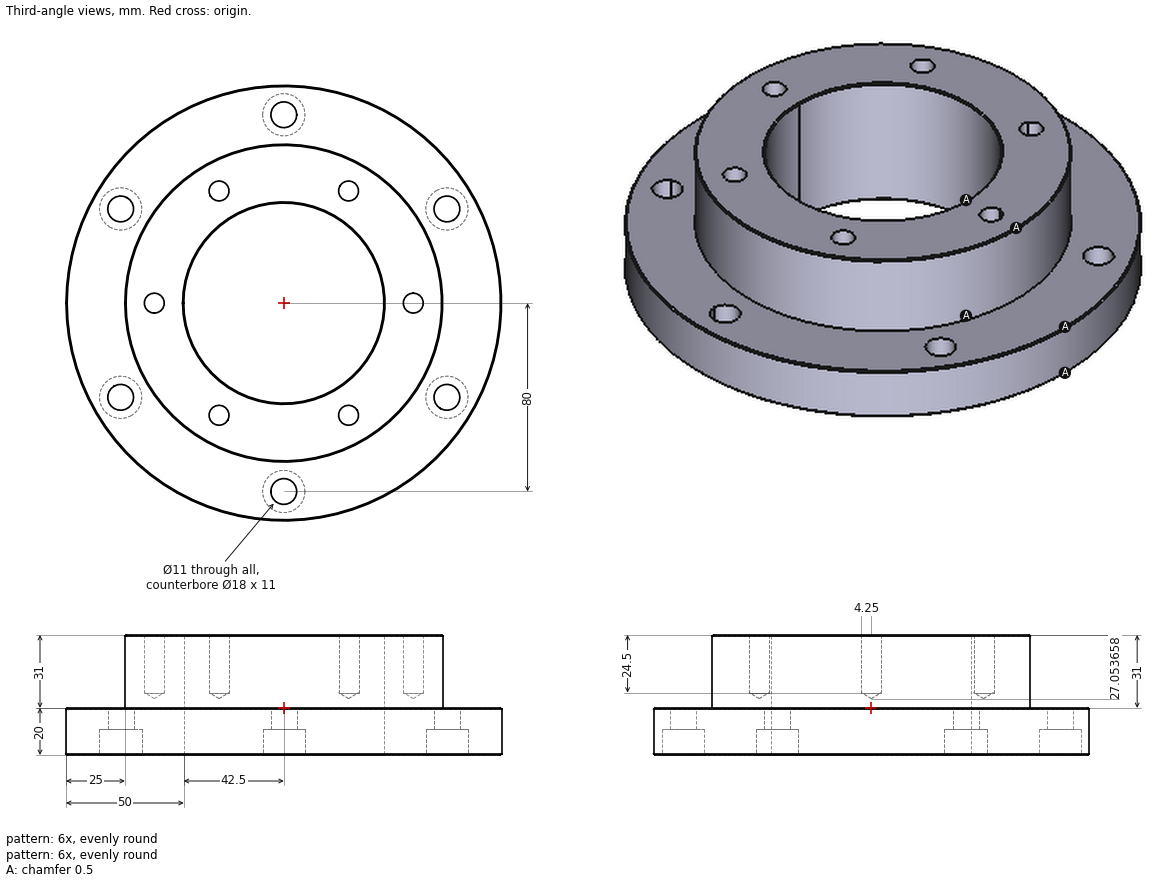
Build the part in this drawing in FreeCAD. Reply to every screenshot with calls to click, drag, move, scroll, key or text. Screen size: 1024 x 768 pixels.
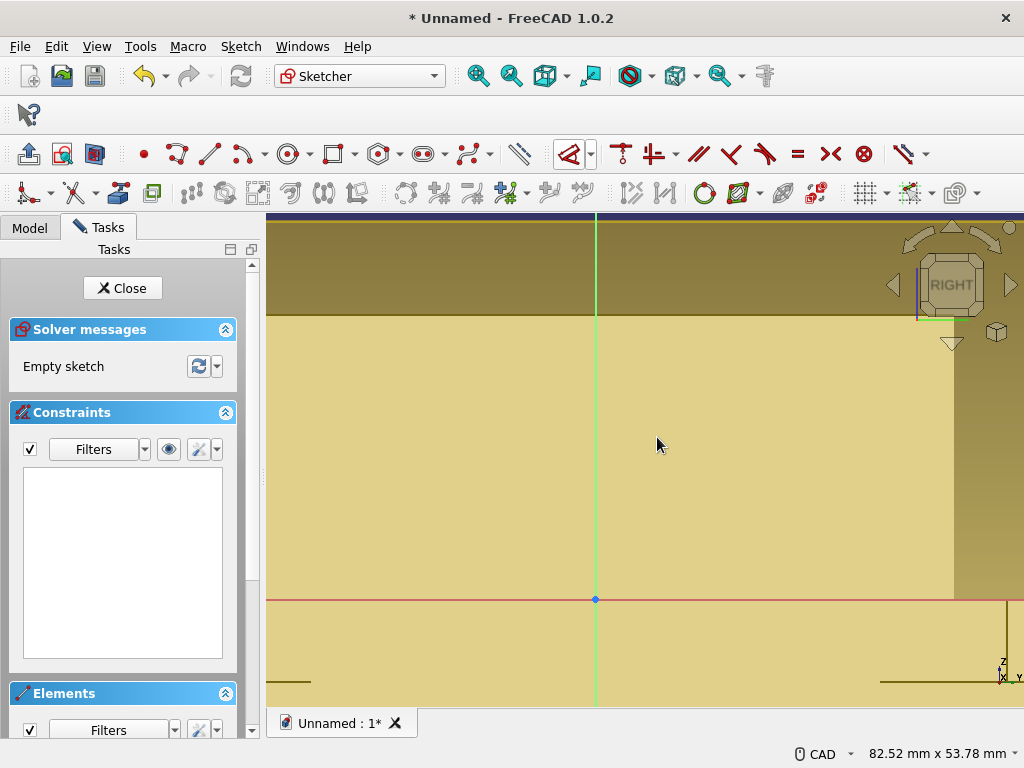
click(177, 154)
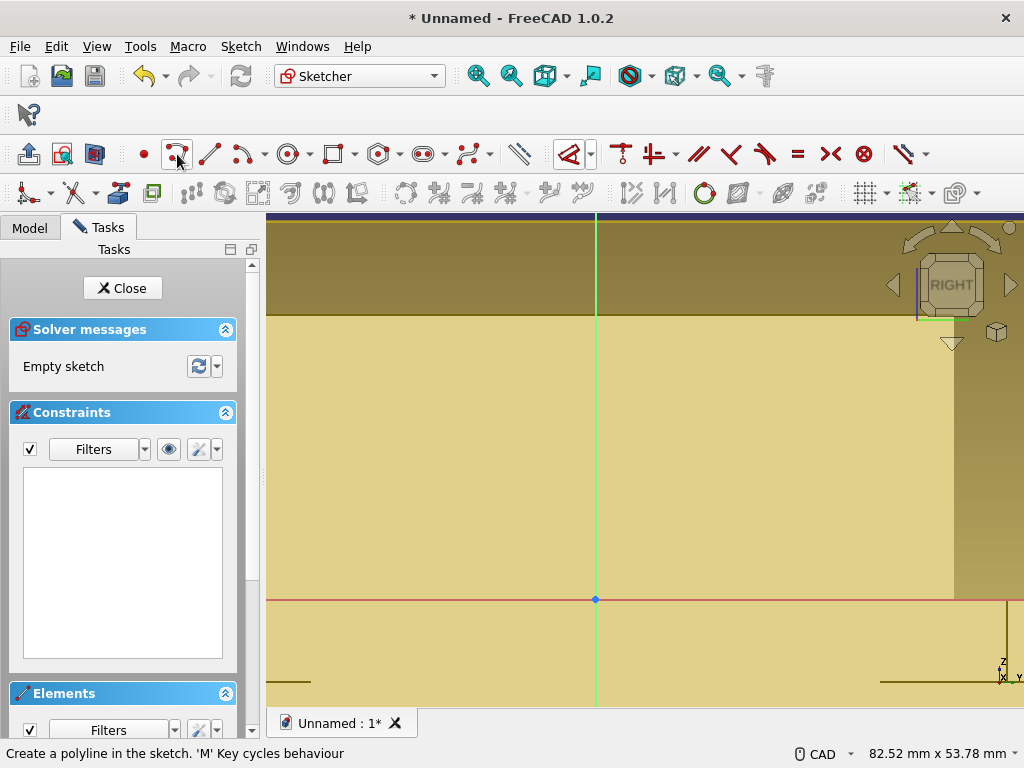
click(596, 563)
click(587, 315)
click(556, 315)
click(556, 540)
click(596, 564)
key(Escape)
key(Escape)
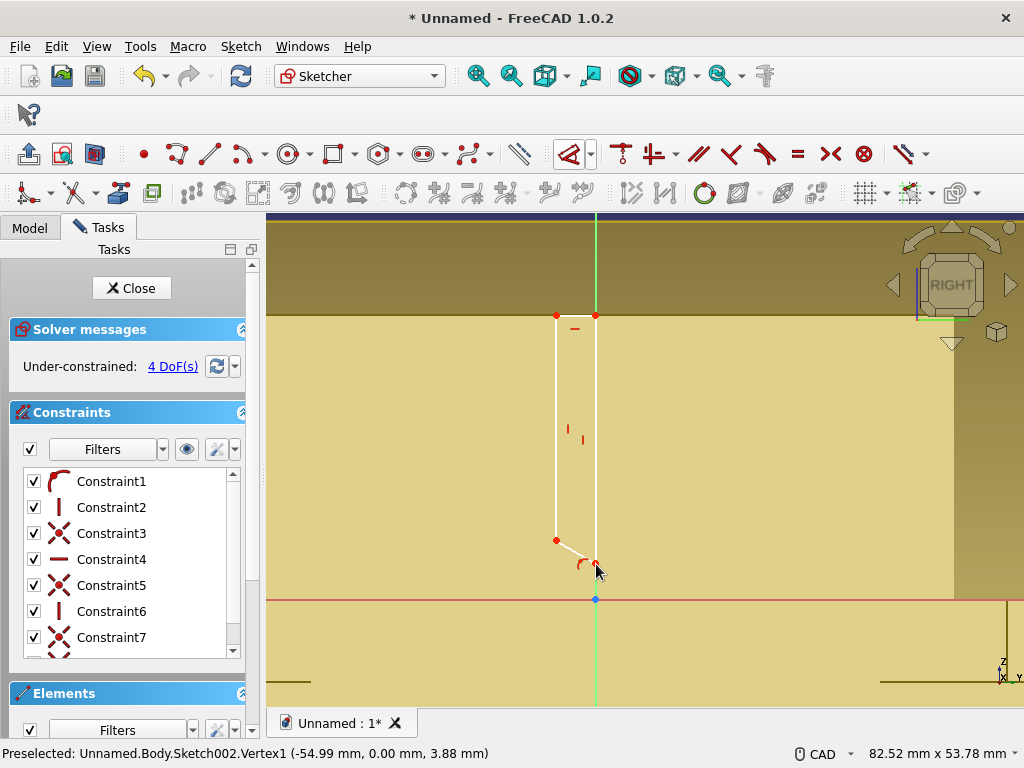
click(596, 316)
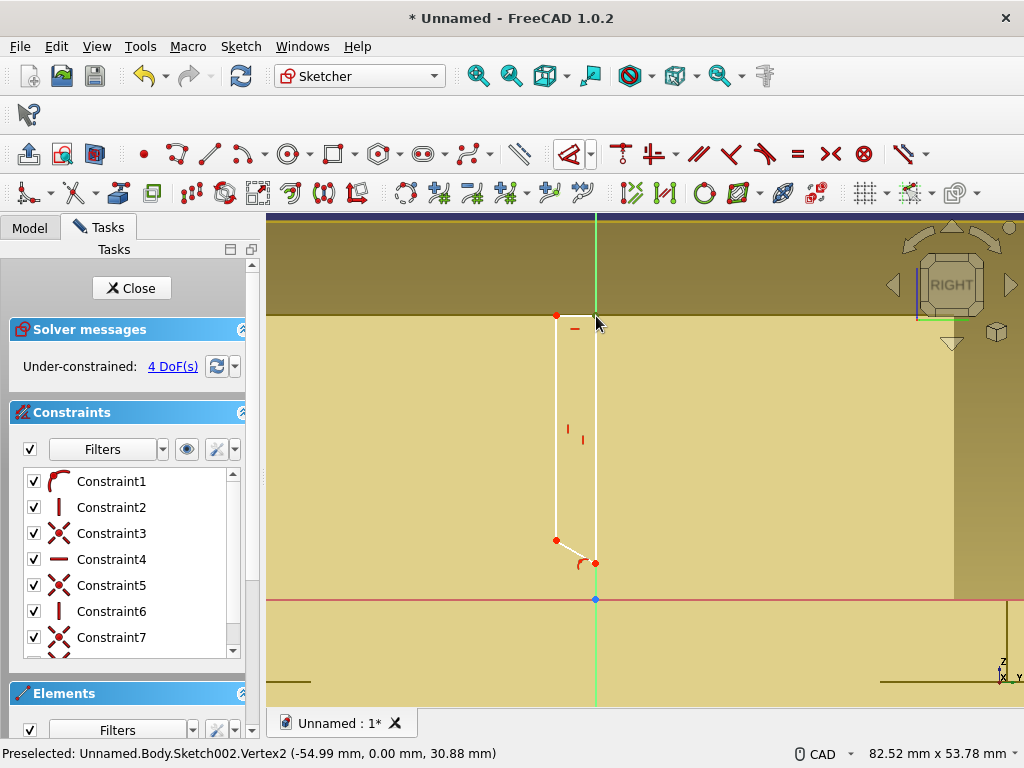
click(590, 154)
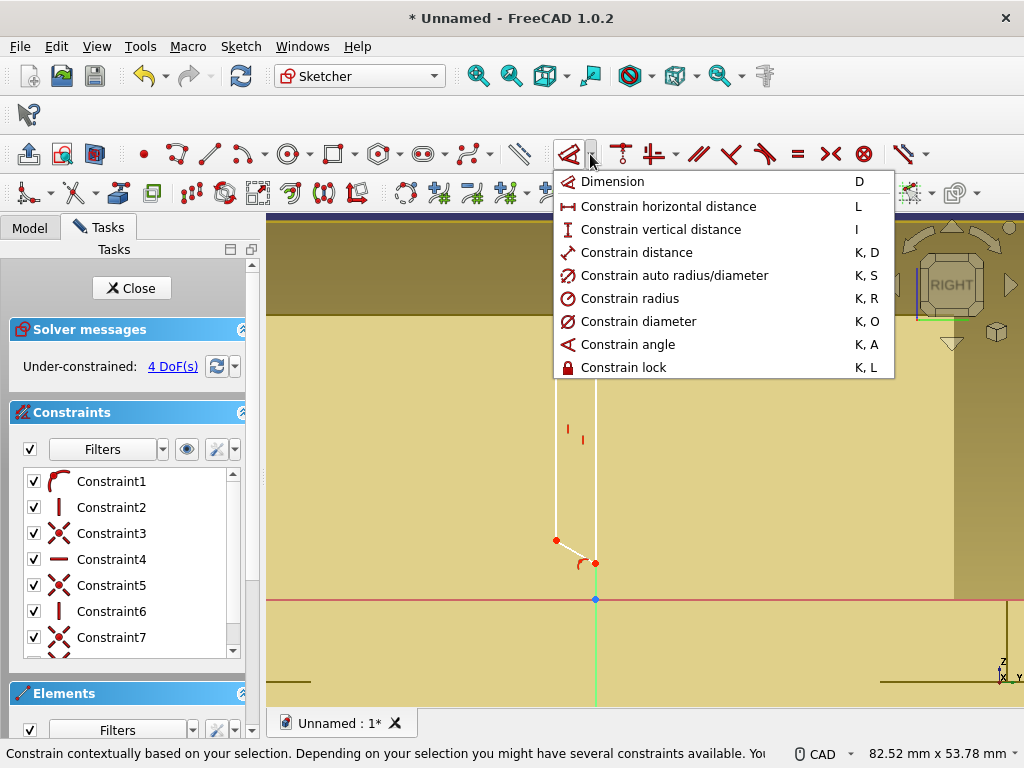
click(724, 230)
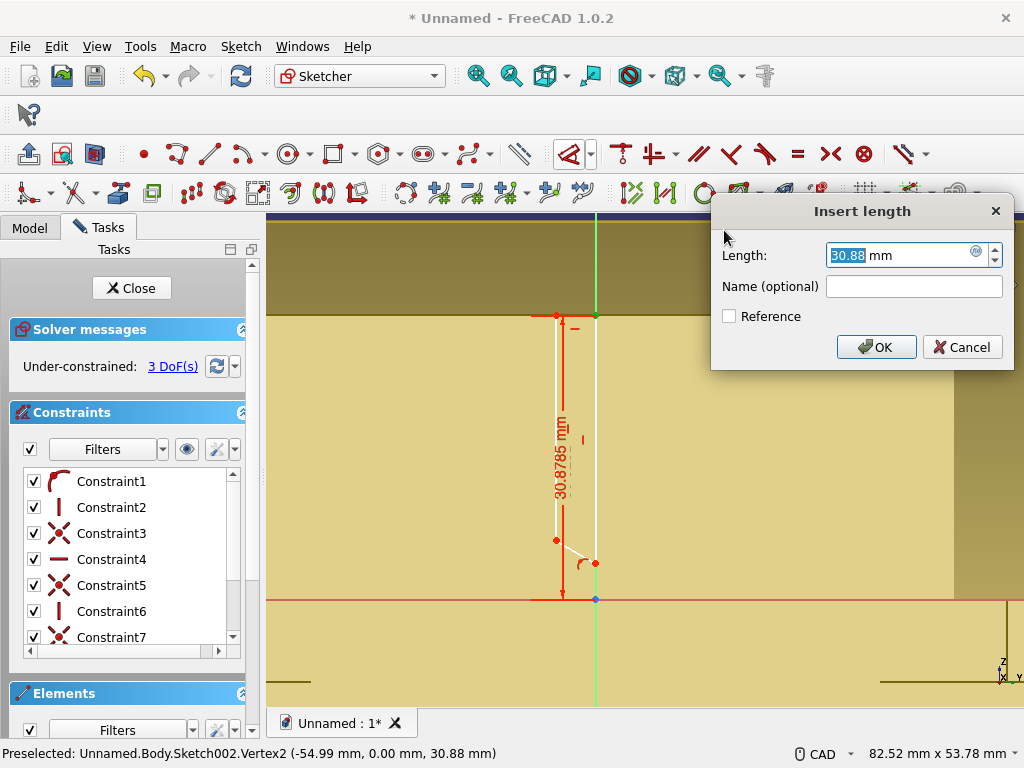
text(31)
key(Return)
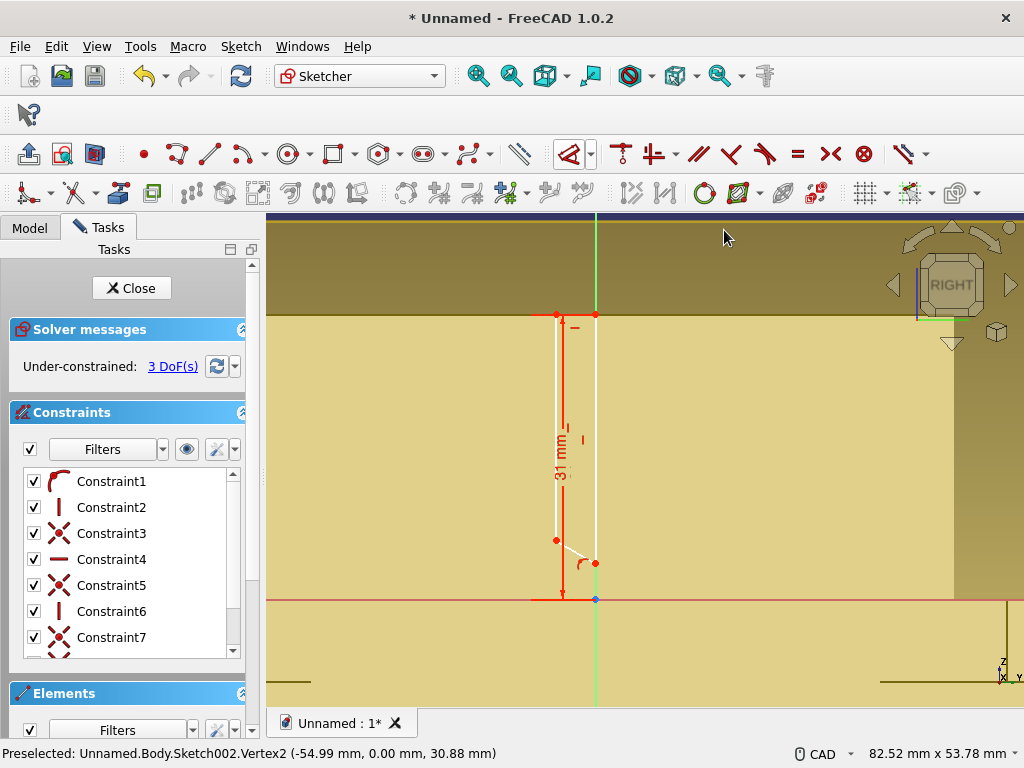
click(584, 315)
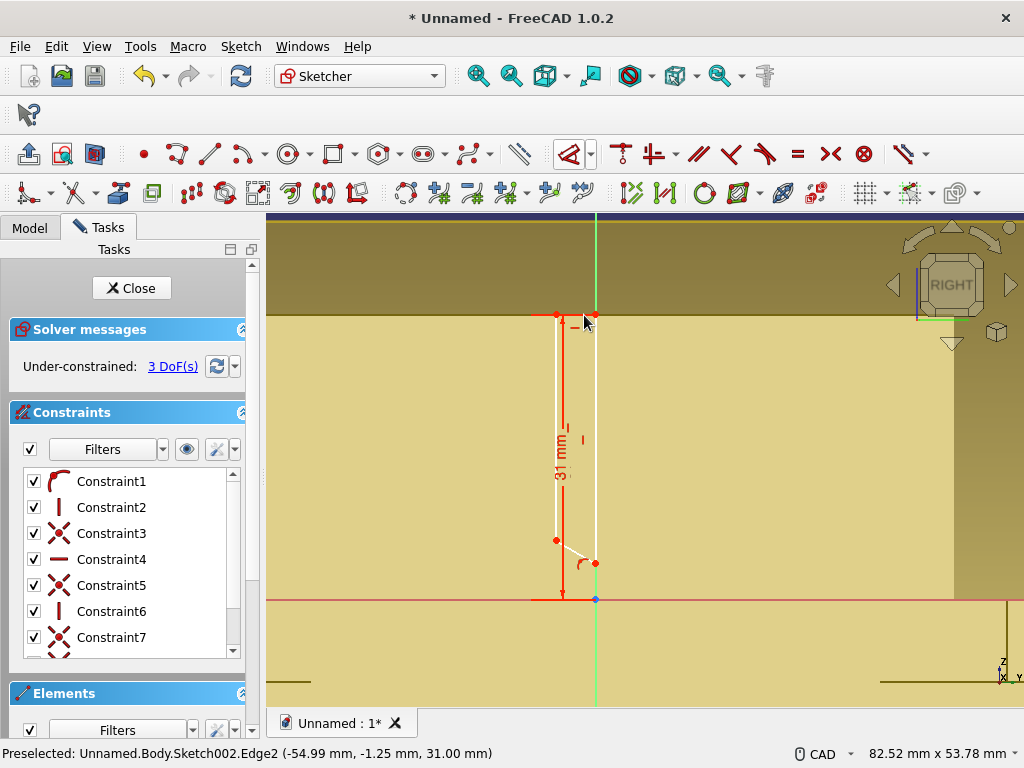
click(590, 154)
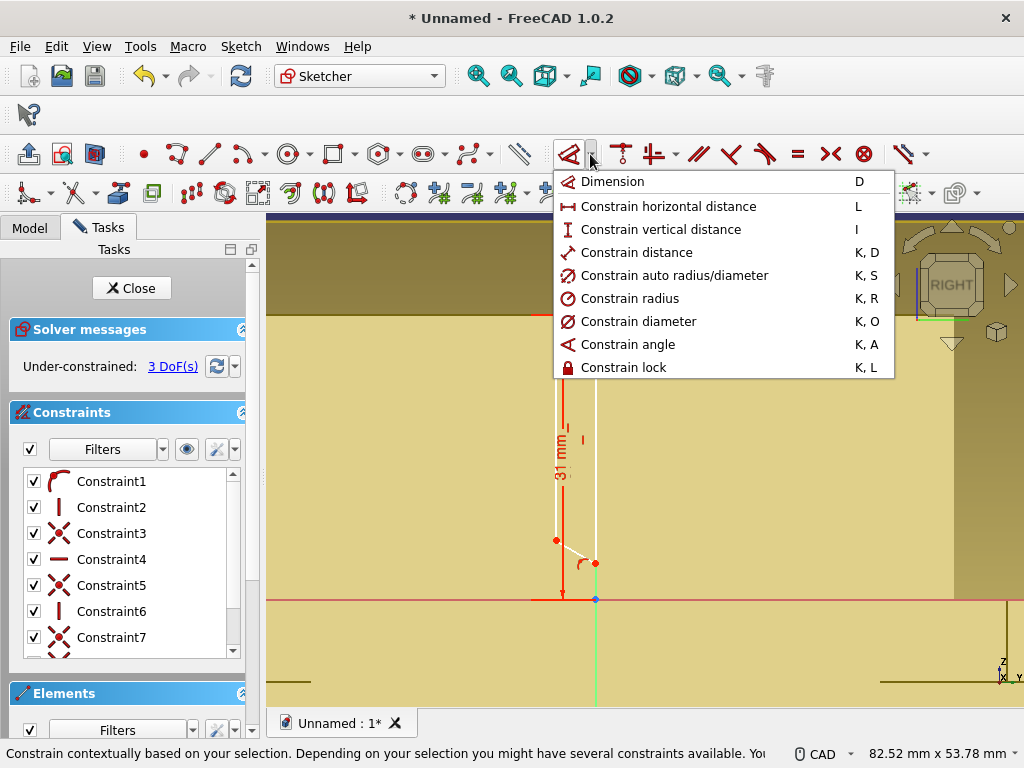
click(724, 206)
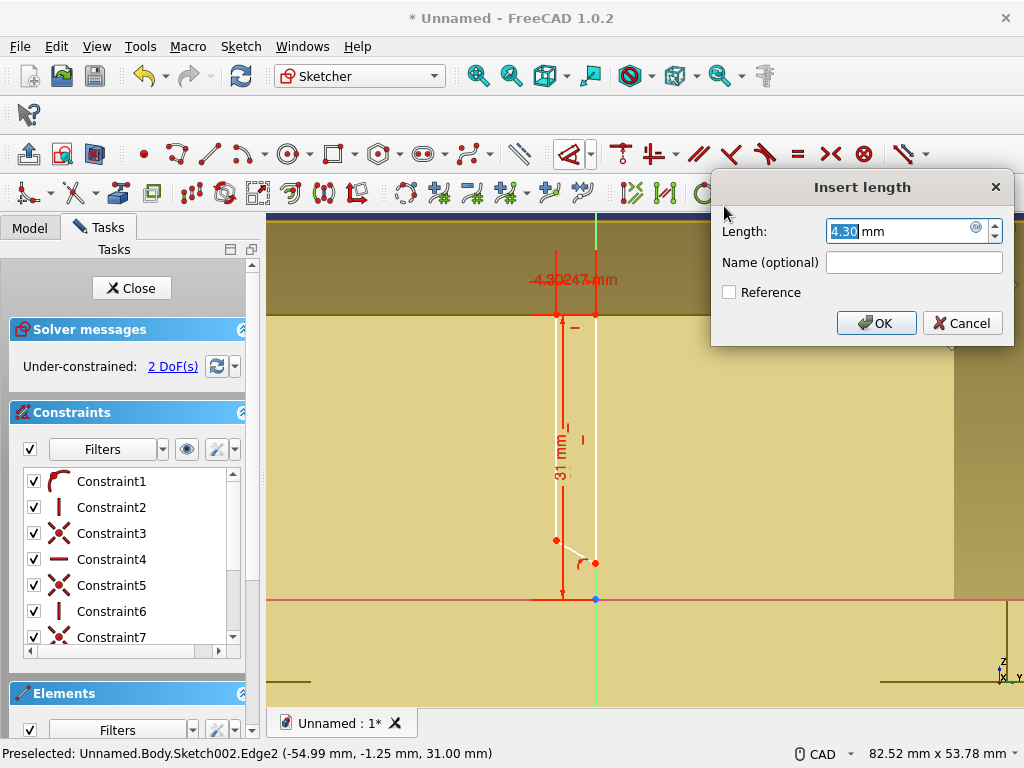
text(4.25)
key(Return)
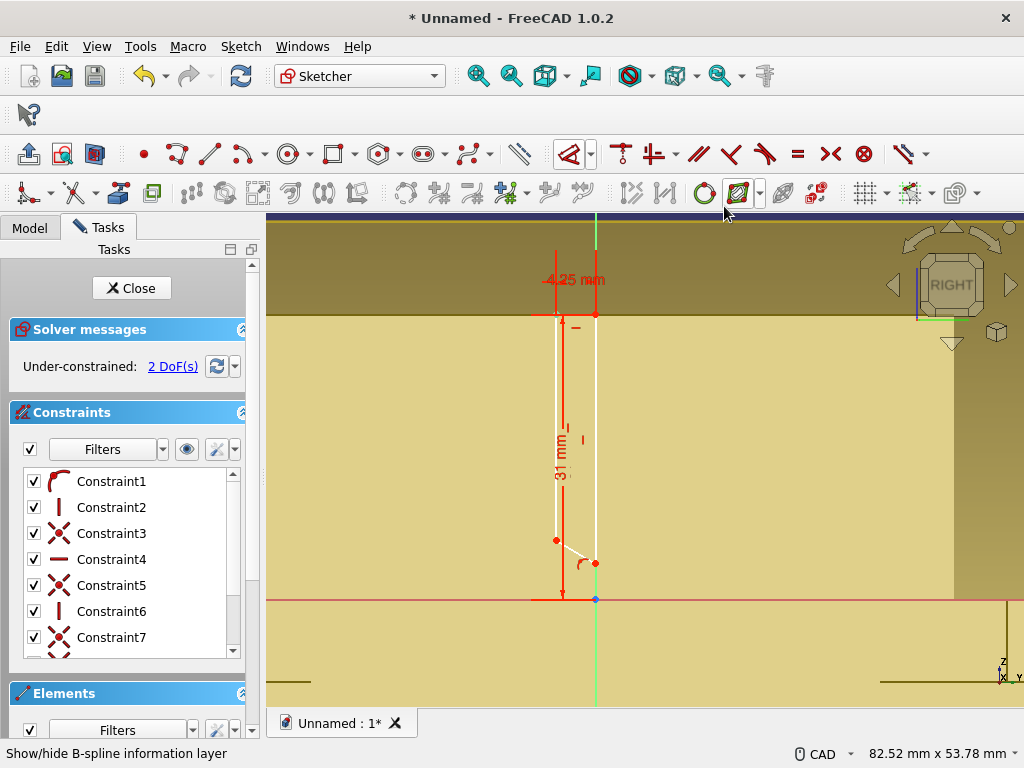
click(556, 383)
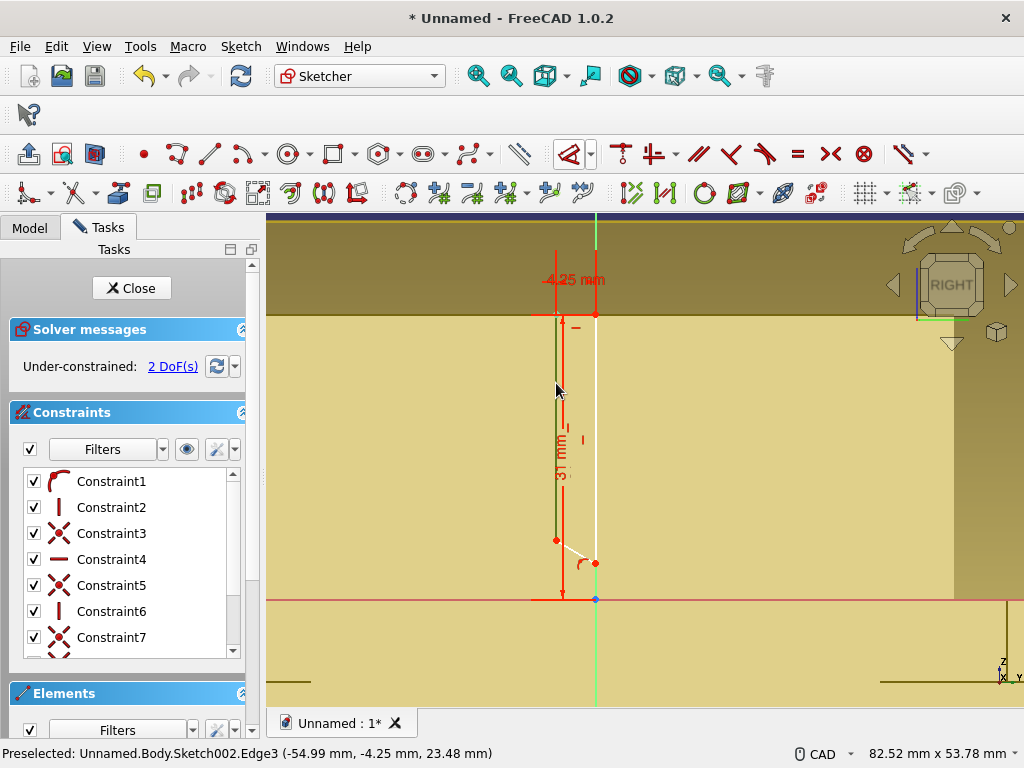
key(i)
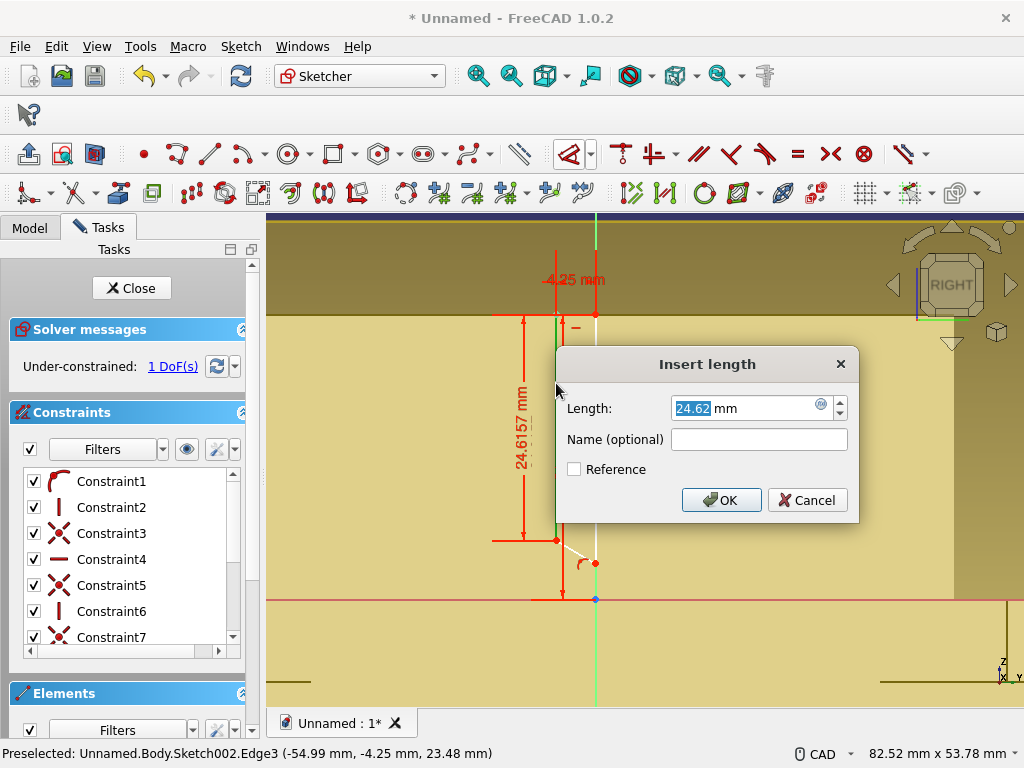
text(24.5)
key(Return)